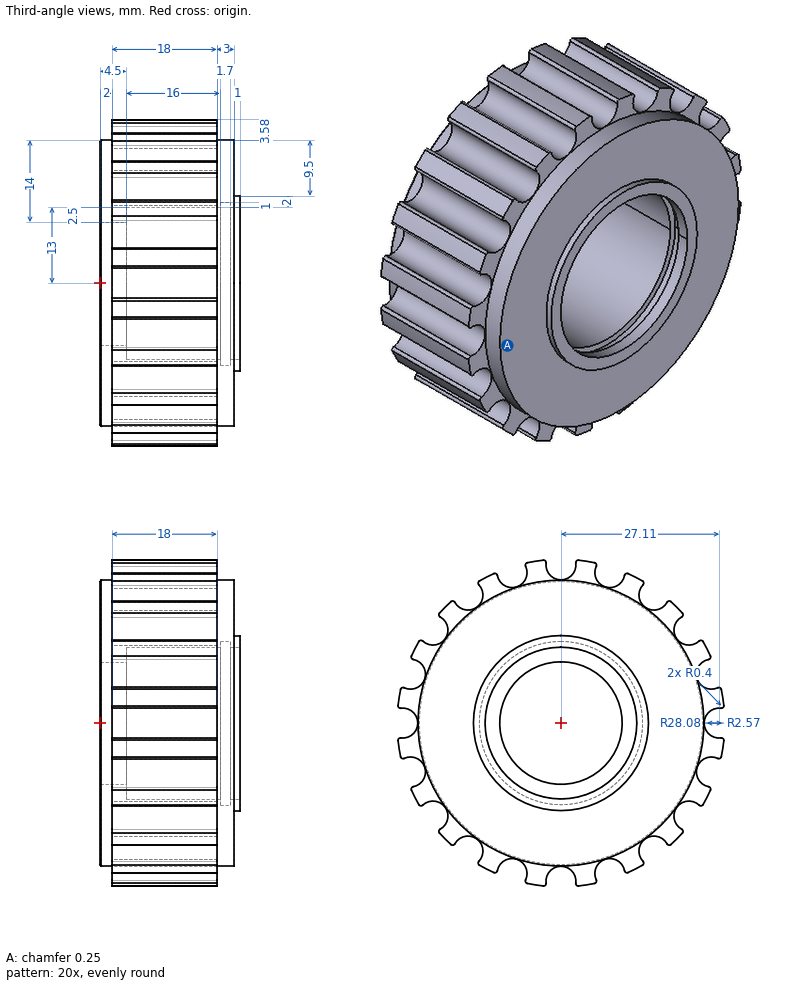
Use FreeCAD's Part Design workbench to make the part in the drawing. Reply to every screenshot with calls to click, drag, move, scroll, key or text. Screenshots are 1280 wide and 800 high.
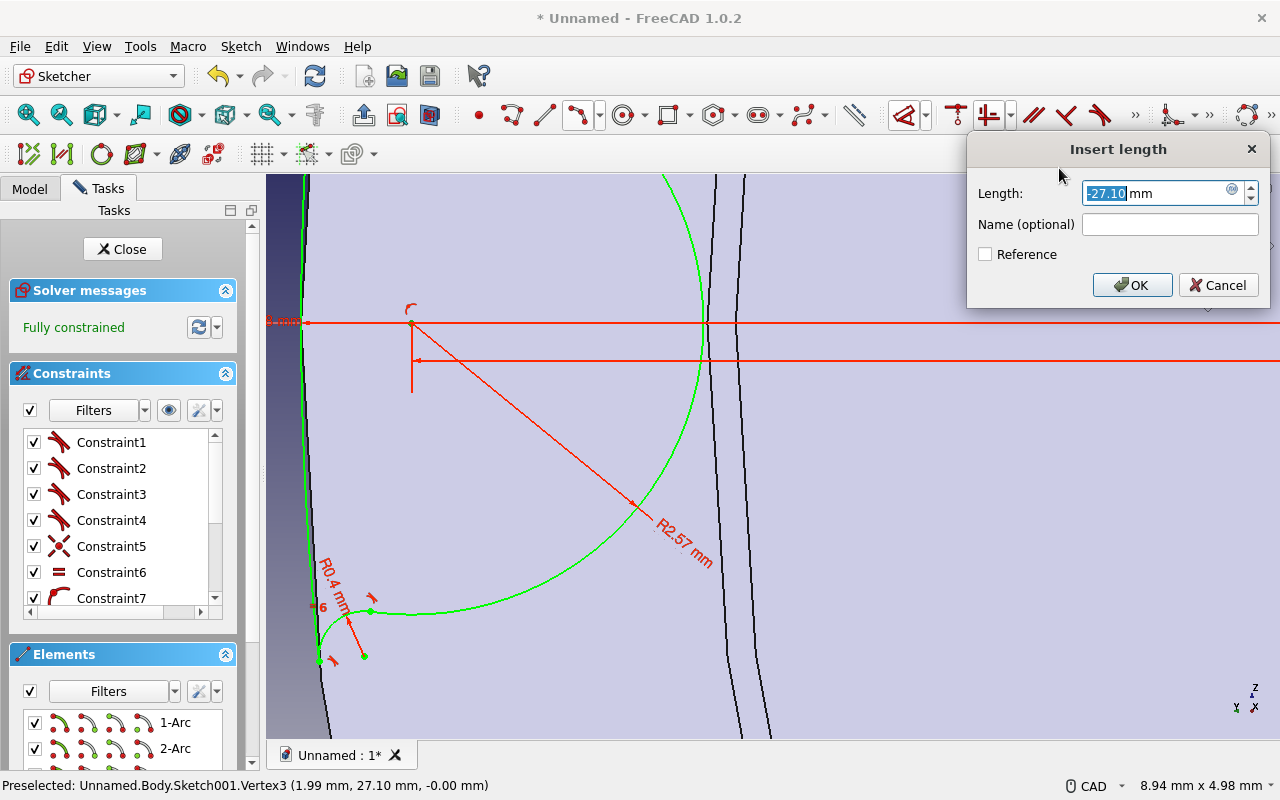
text(-27.11)
key(Return)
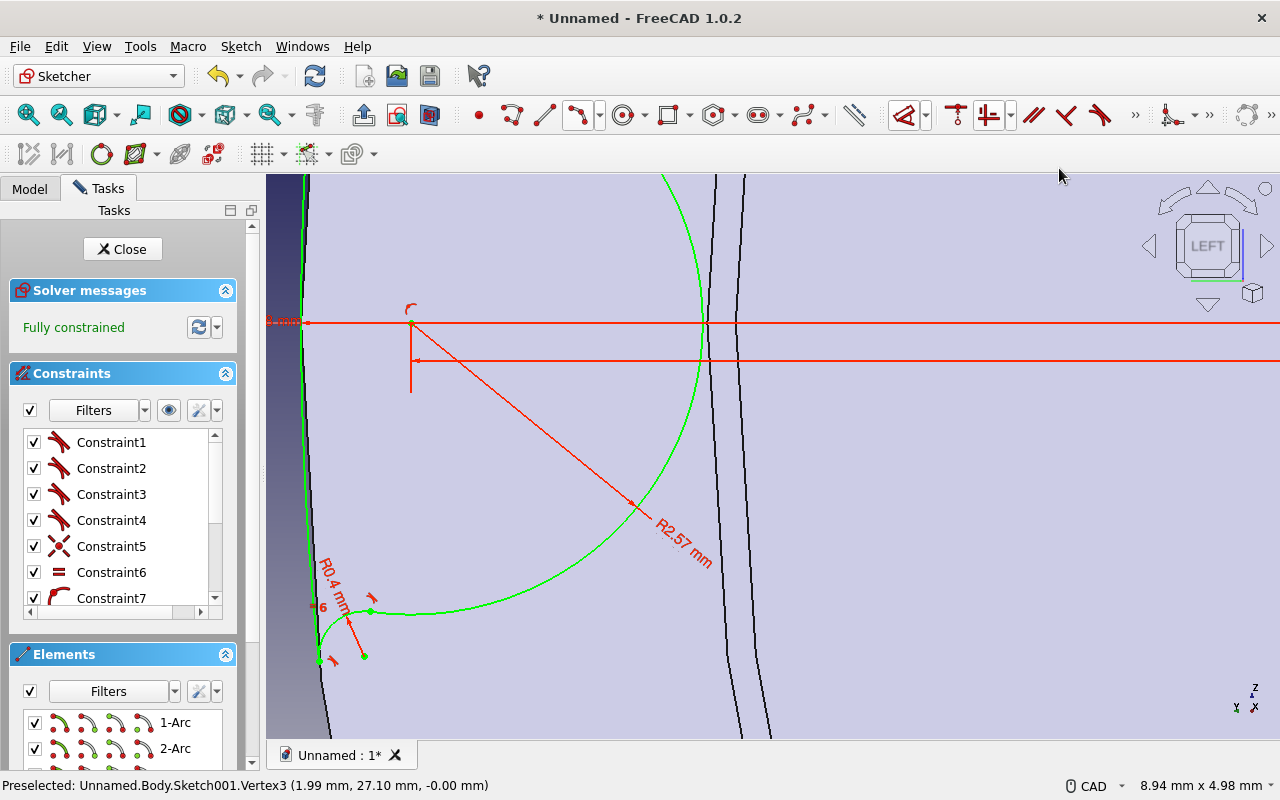
click(123, 249)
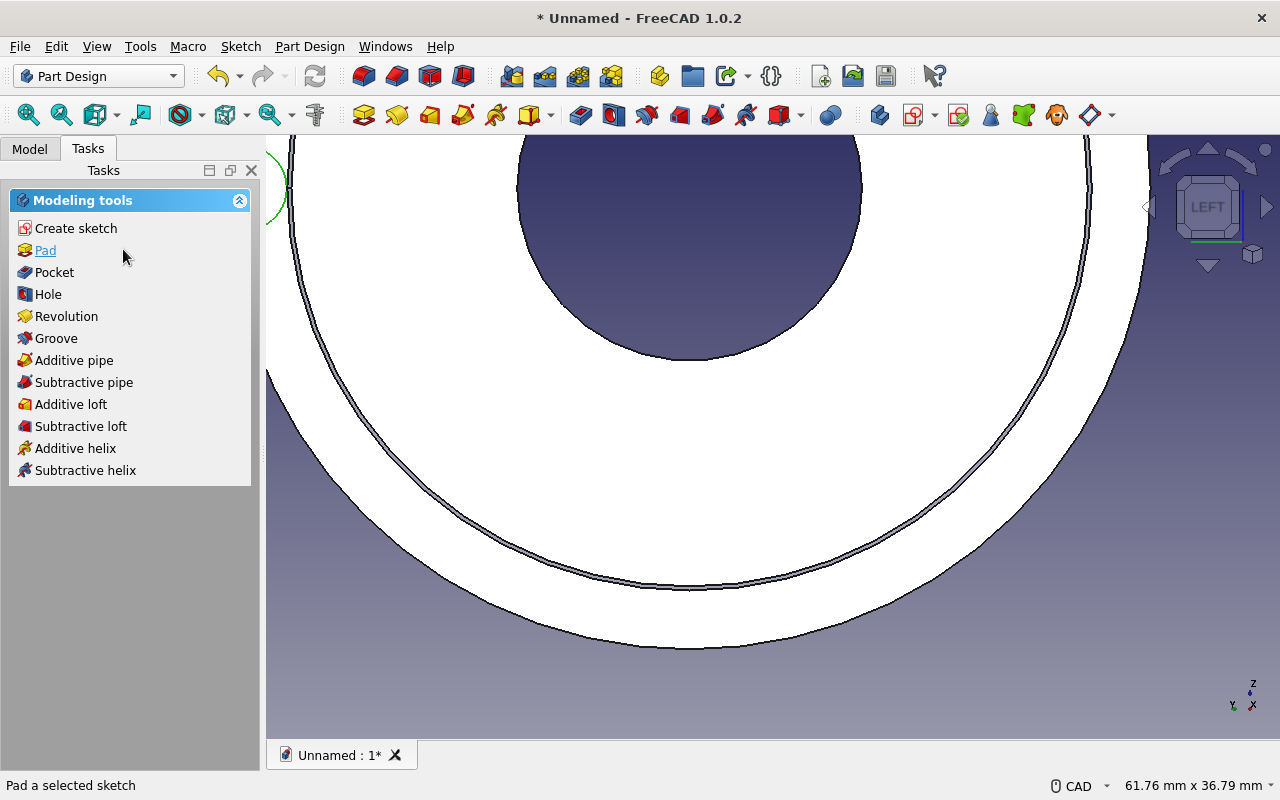
click(581, 116)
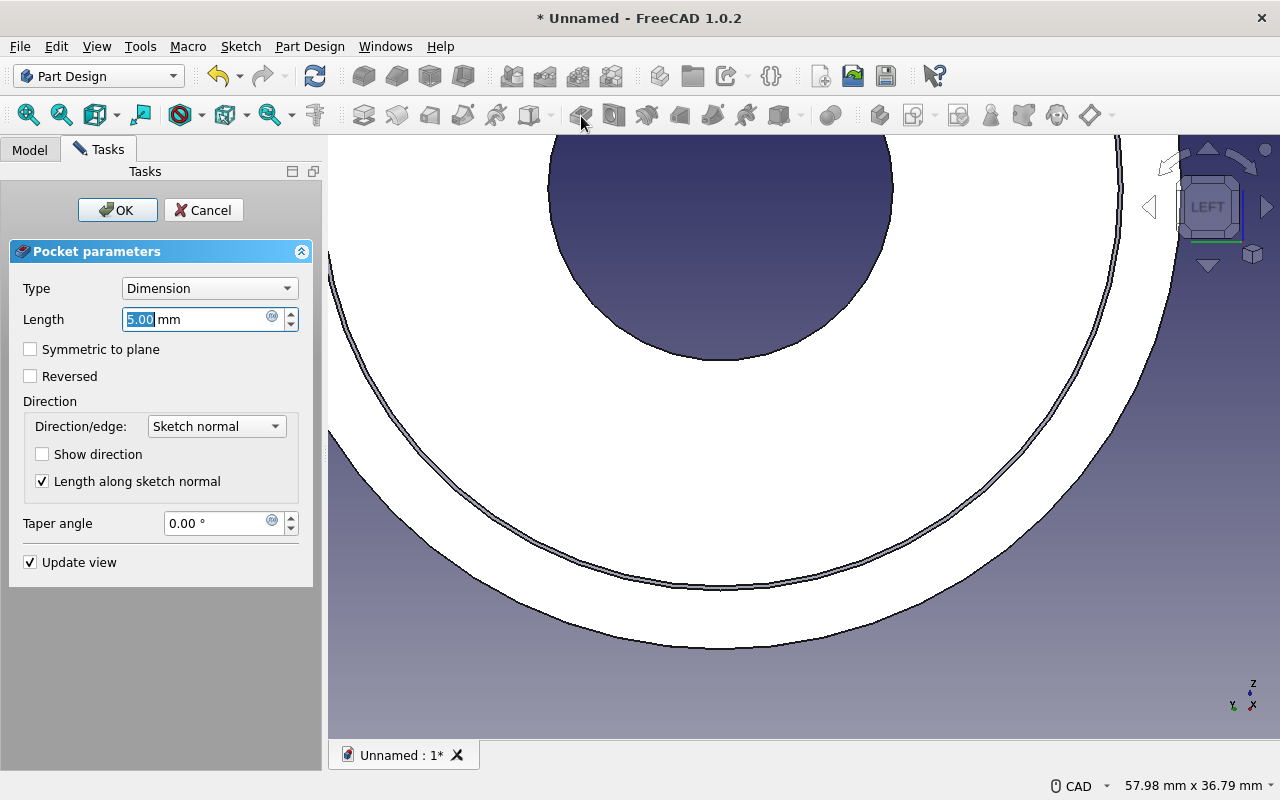
text(18)
key(Tab)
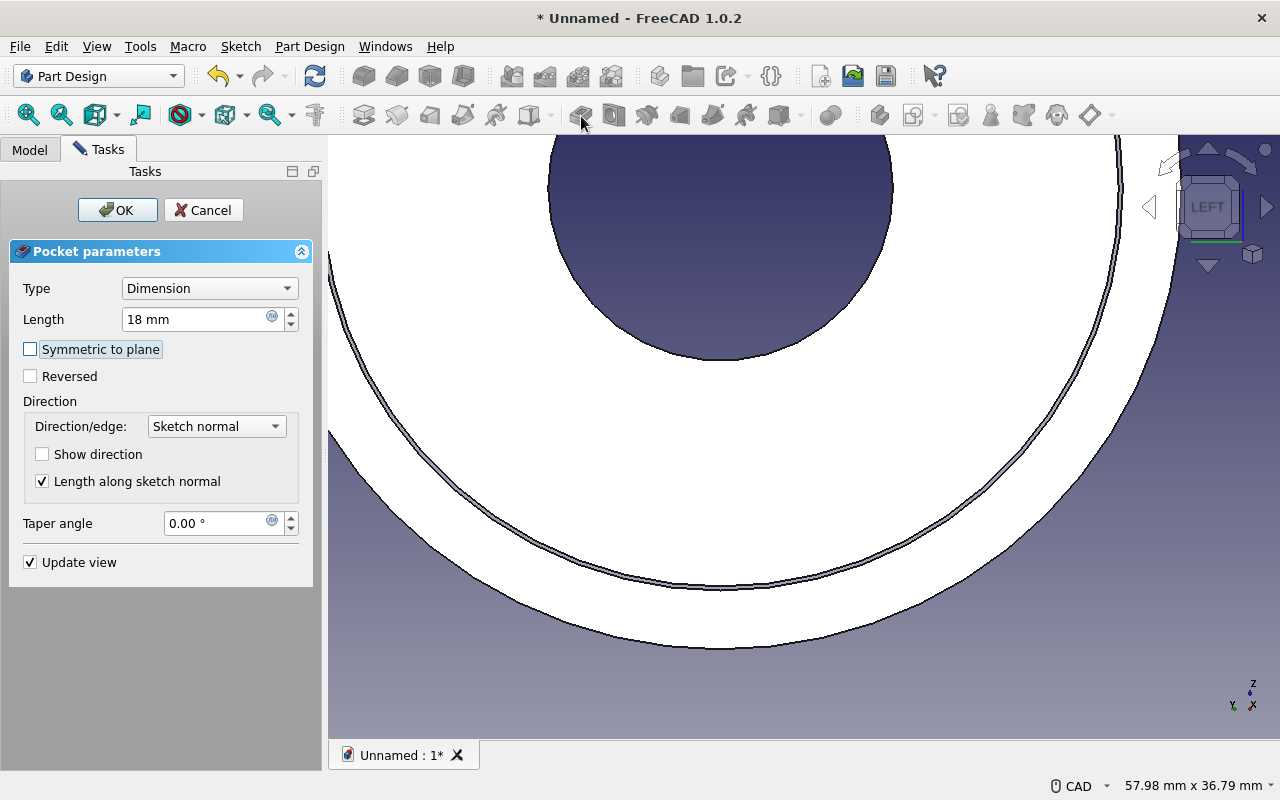
click(118, 210)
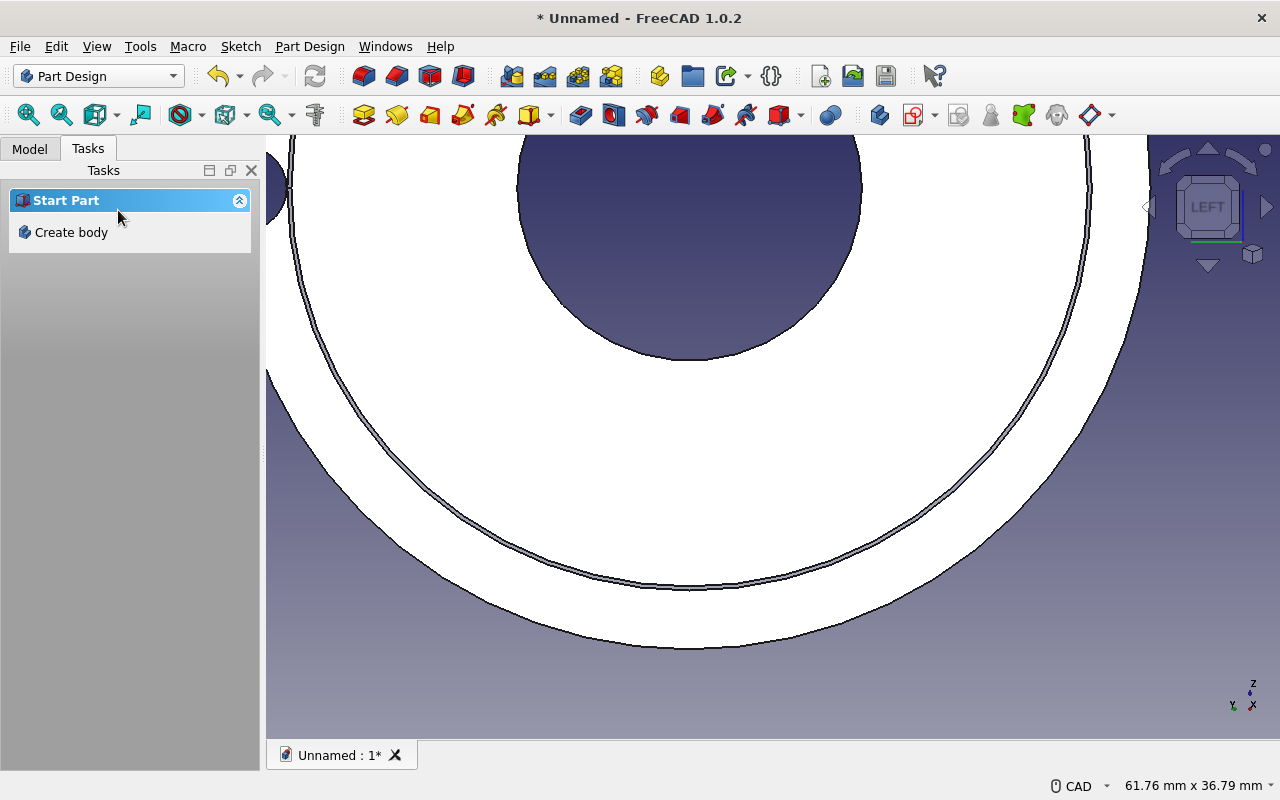
click(29, 116)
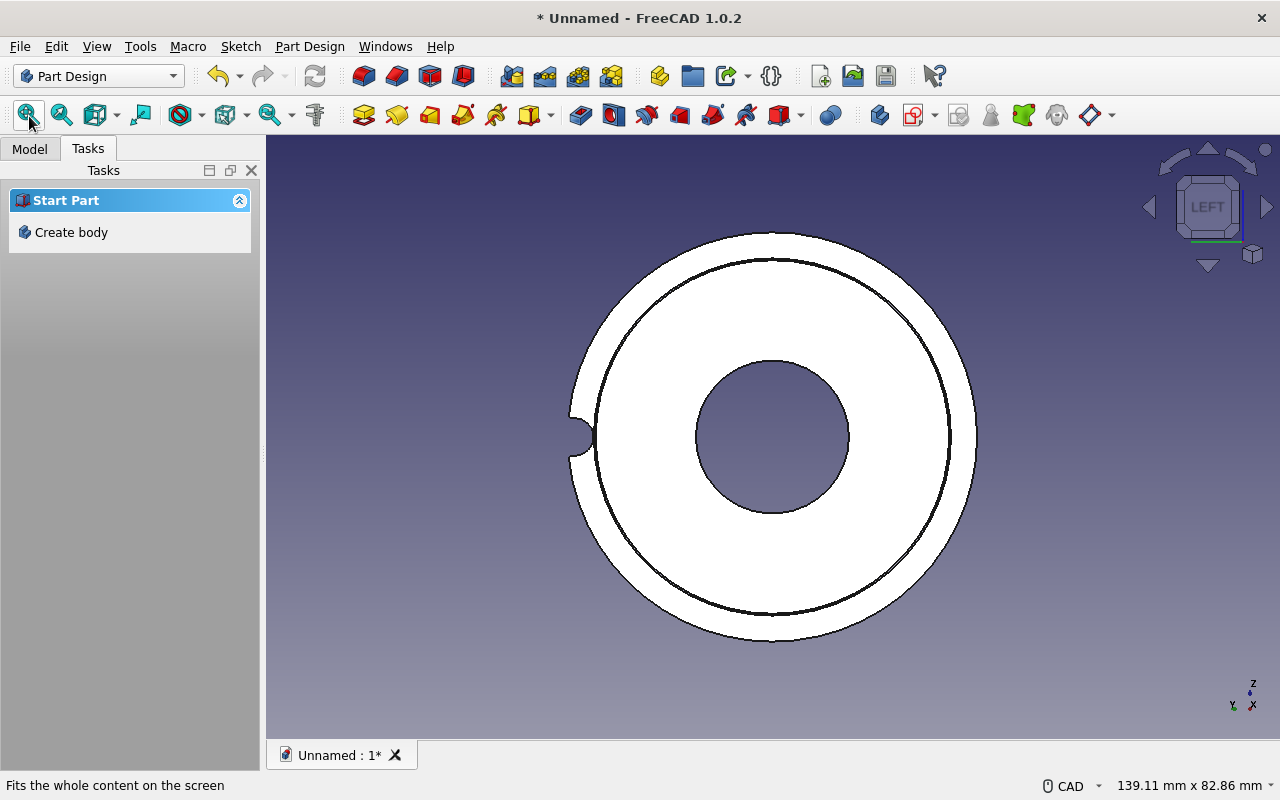
click(30, 148)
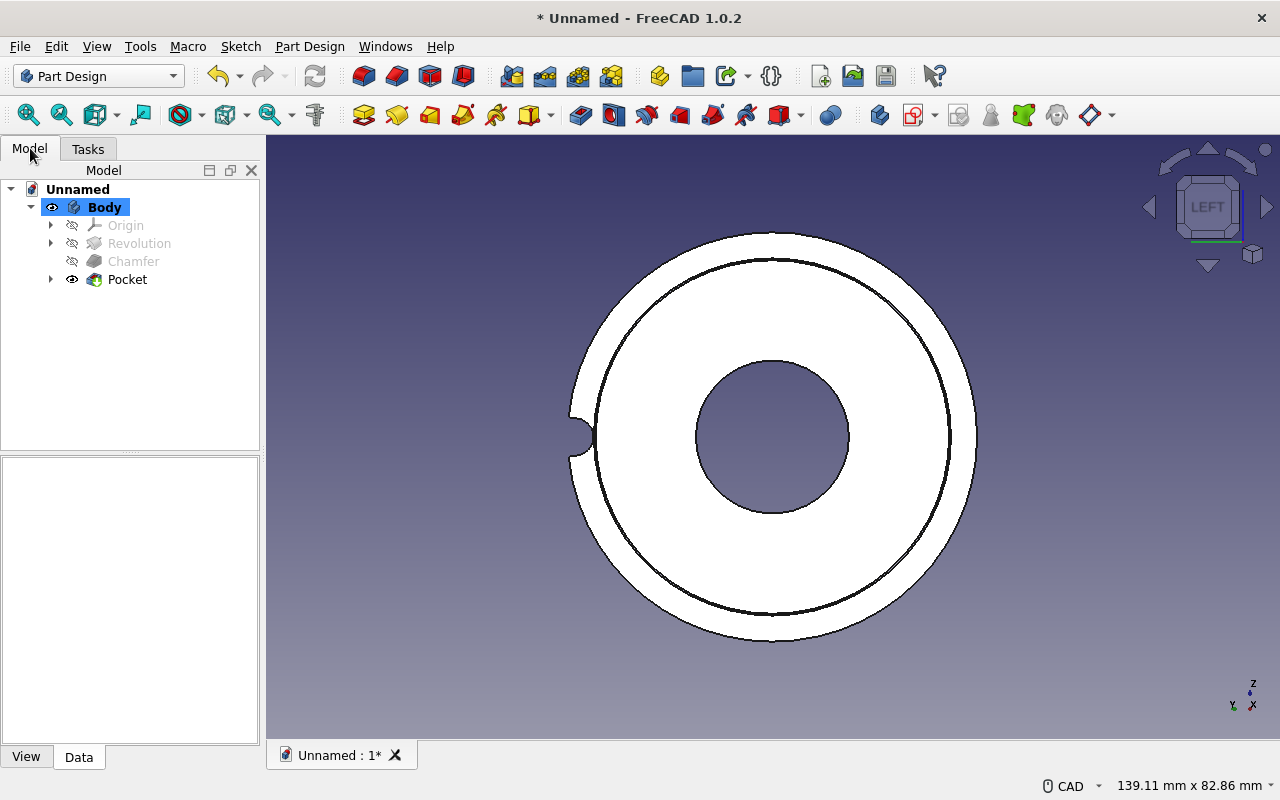
click(117, 279)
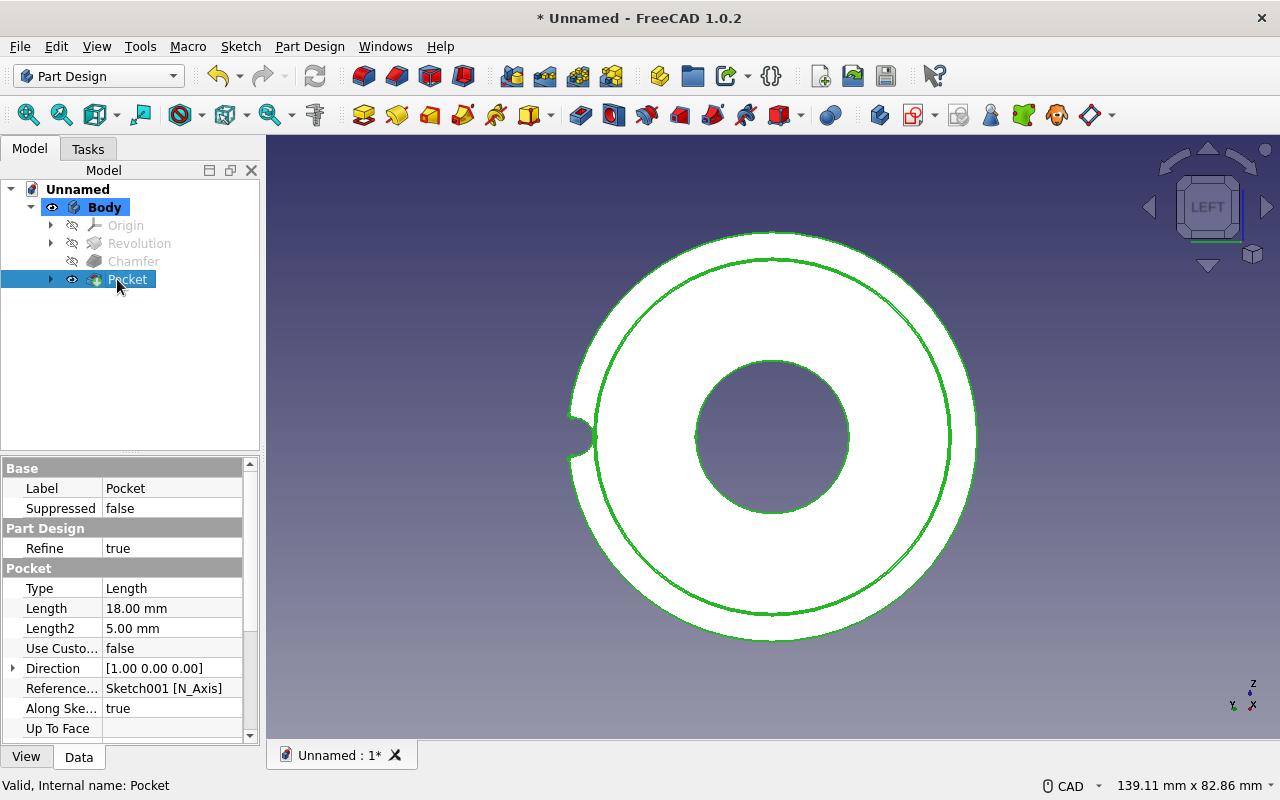
click(578, 76)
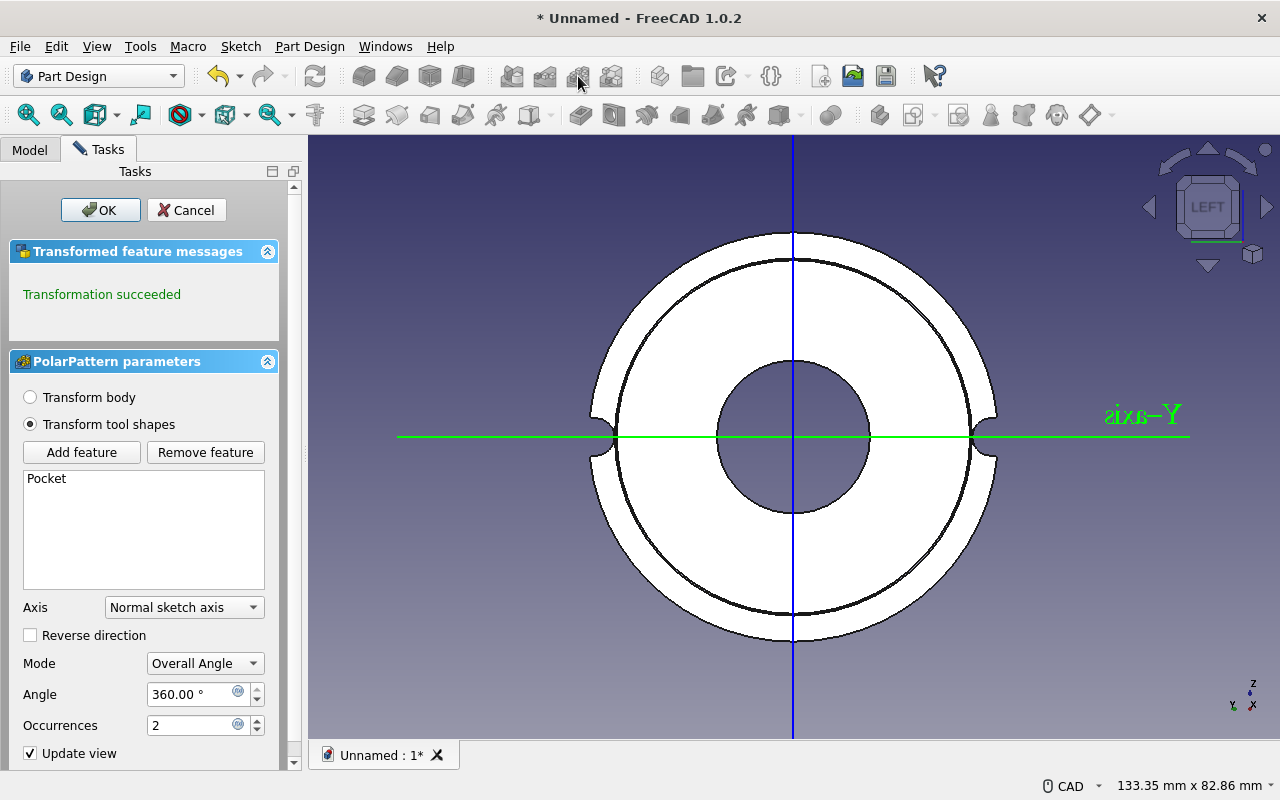
click(185, 608)